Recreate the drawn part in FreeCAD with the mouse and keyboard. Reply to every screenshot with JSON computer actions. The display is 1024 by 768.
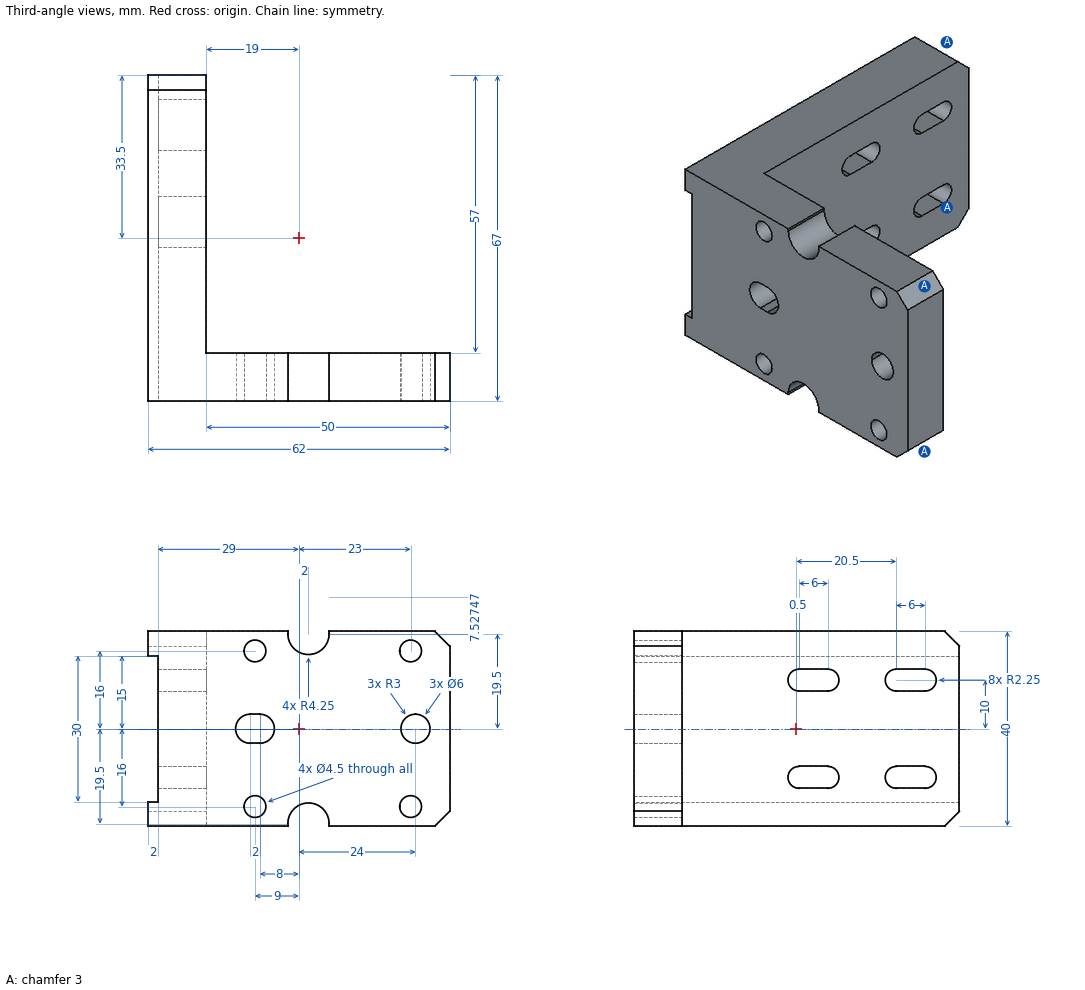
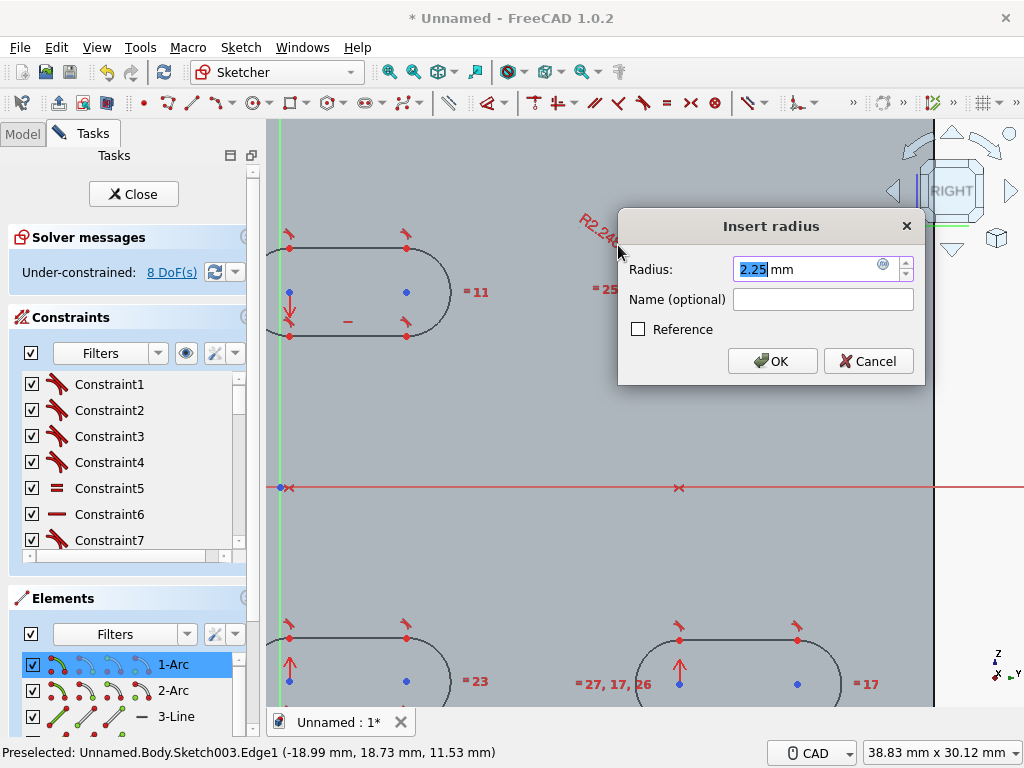
{"action": "type", "text": "2.25"}
{"action": "key", "text": "Return"}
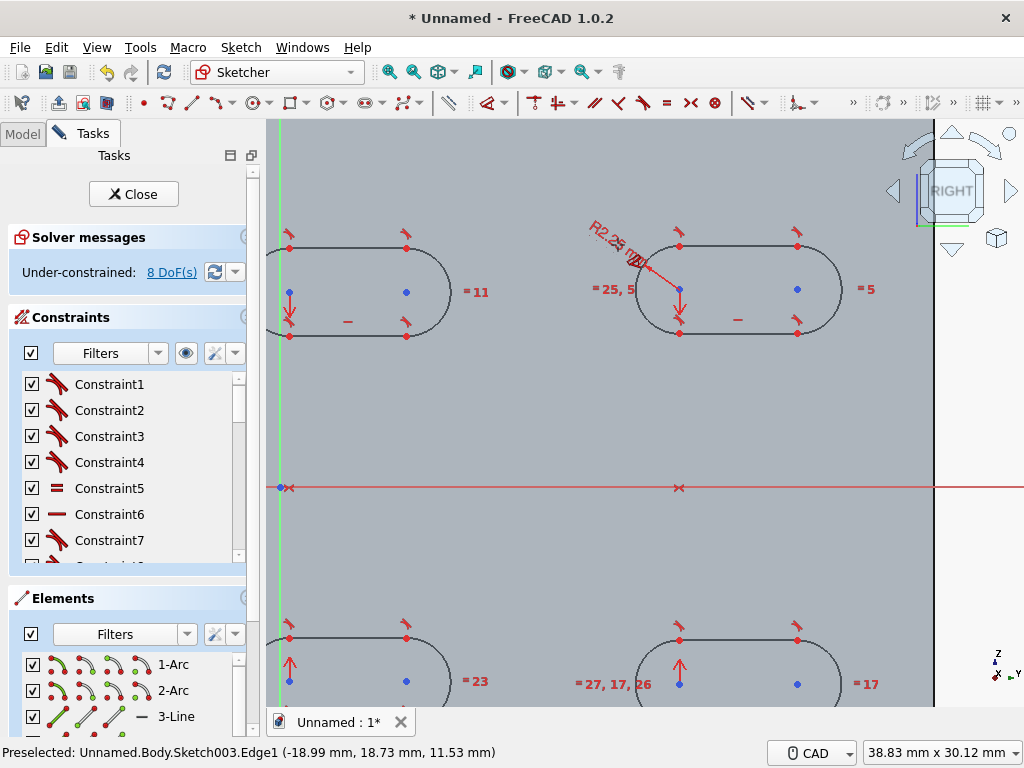
{"action": "left_click", "coordinate": [715, 246]}
{"action": "left_click", "coordinate": [739, 212]}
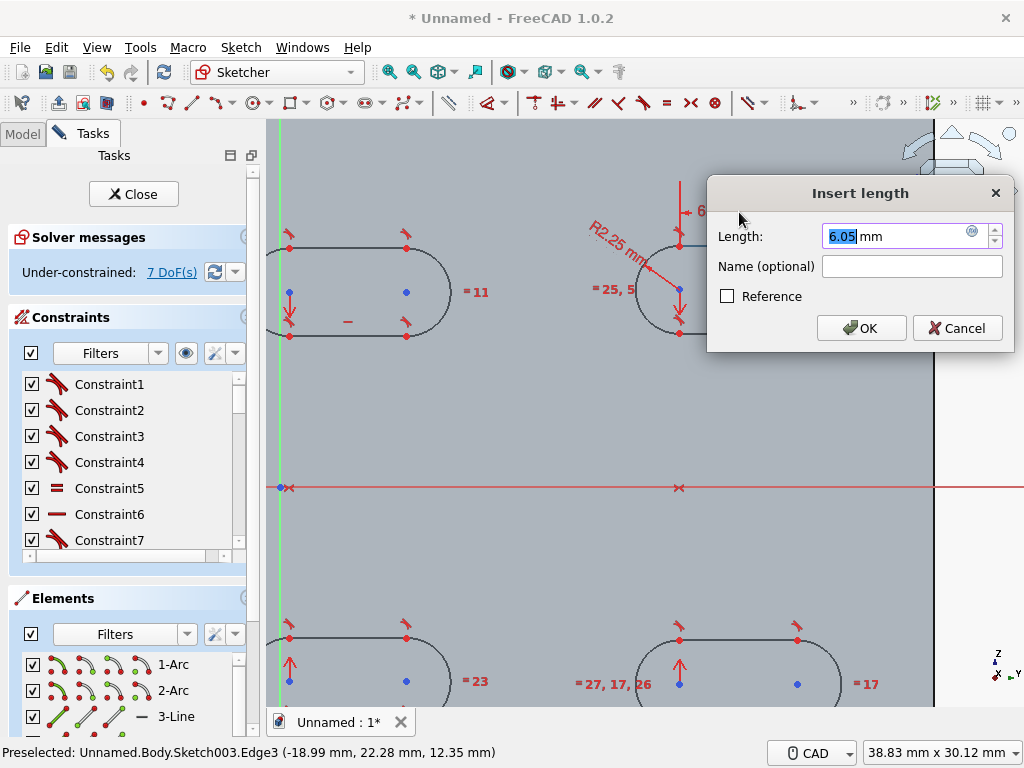
{"action": "type", "text": "6"}
{"action": "key", "text": "Return"}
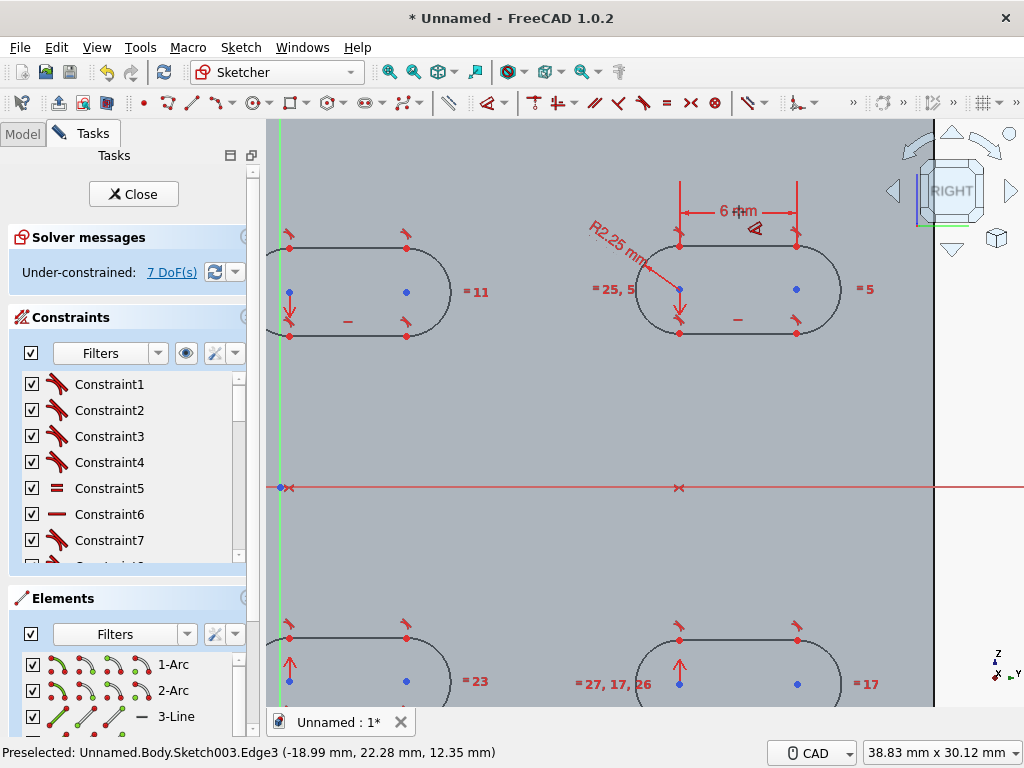
{"action": "left_click", "coordinate": [325, 248]}
{"action": "left_click", "coordinate": [350, 214]}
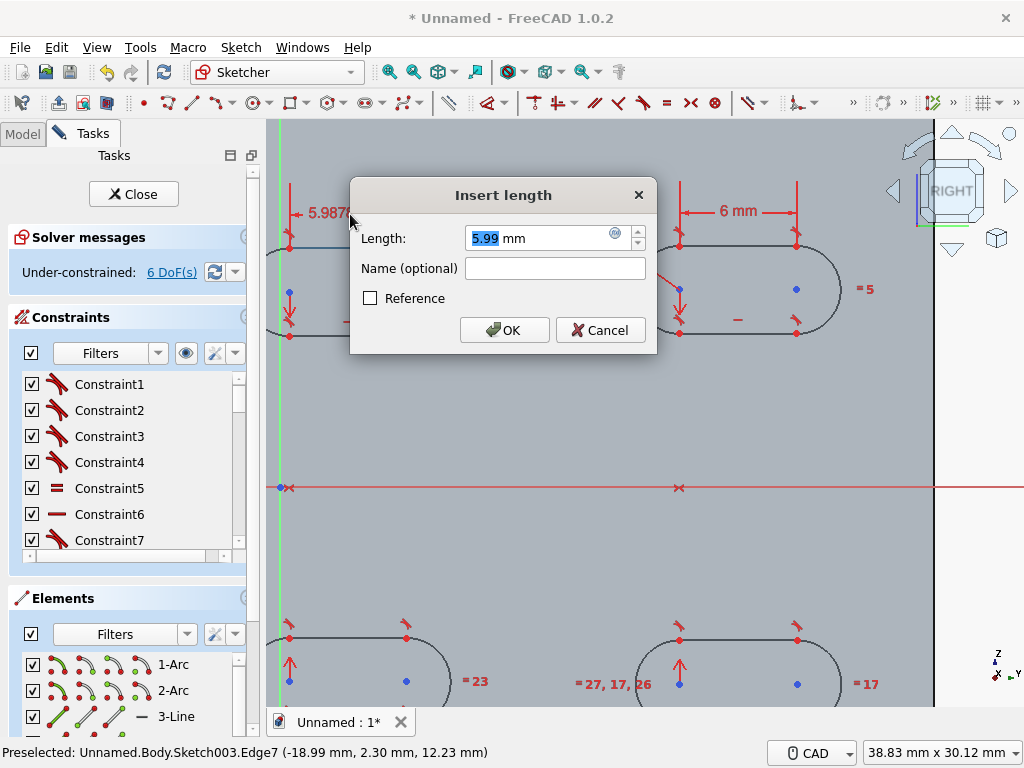
{"action": "type", "text": "6"}
{"action": "key", "text": "Return"}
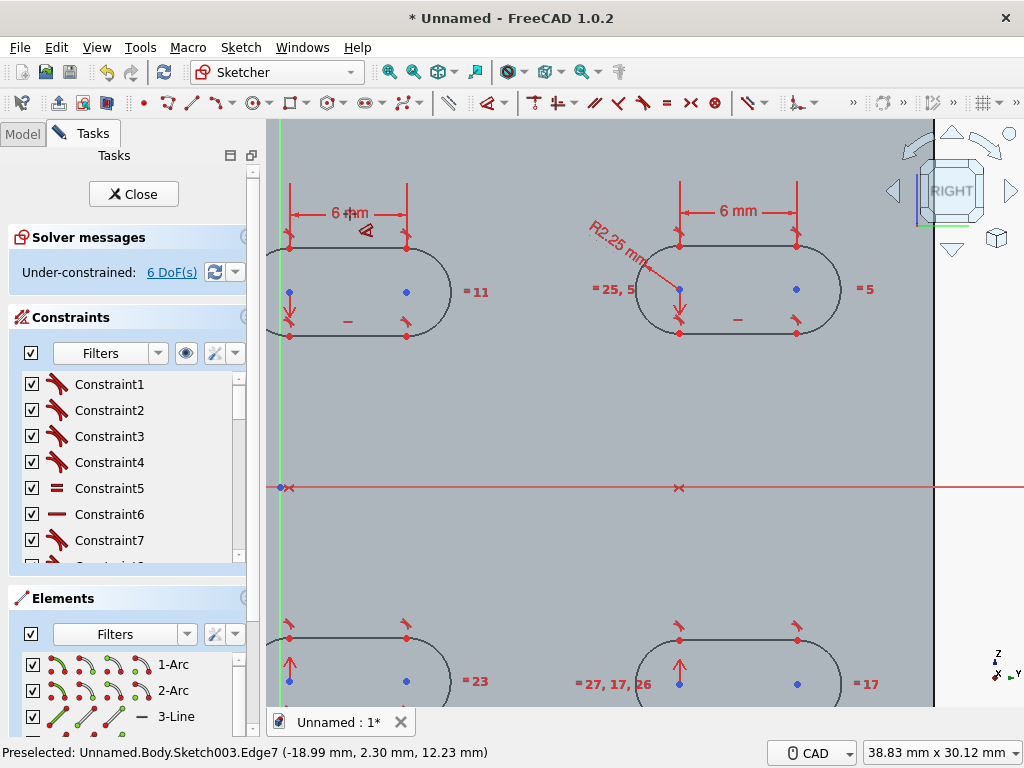
{"action": "left_click", "coordinate": [715, 640]}
{"action": "left_click", "coordinate": [739, 674]}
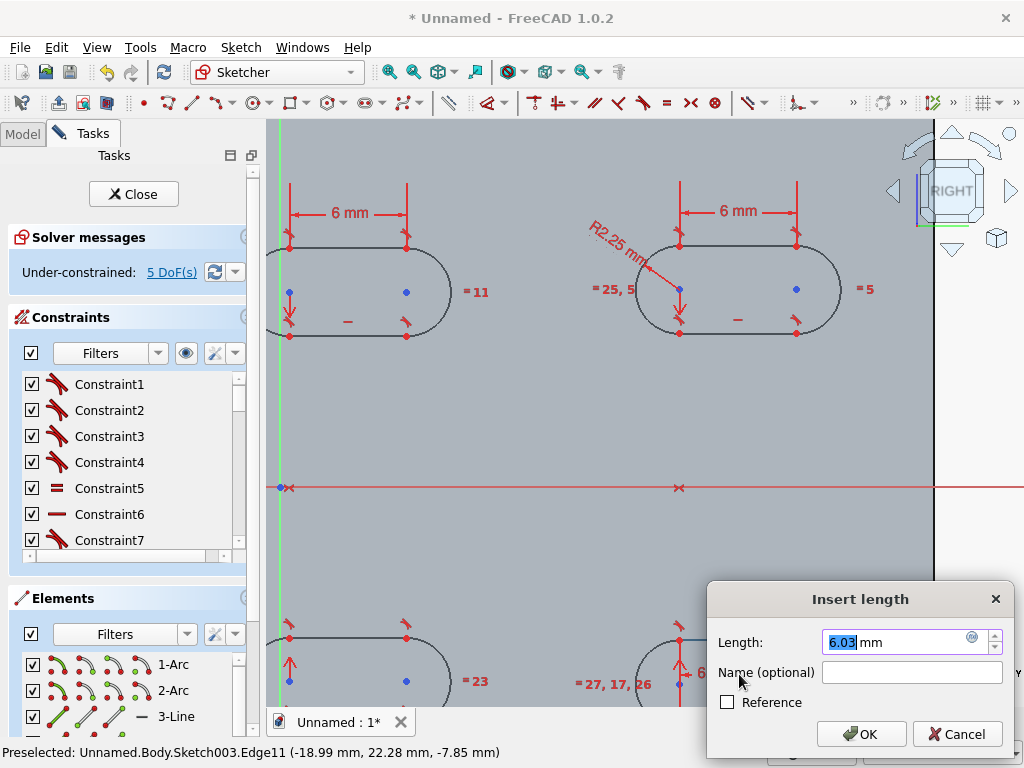
{"action": "type", "text": "6"}
{"action": "key", "text": "Return"}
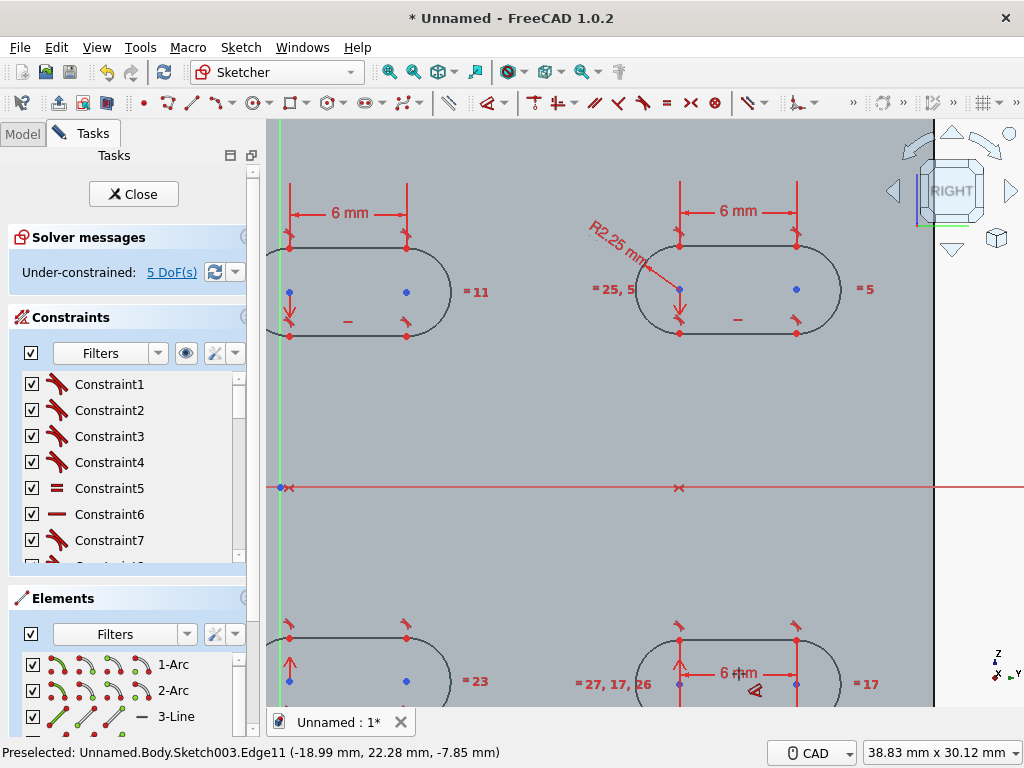
{"action": "left_click", "coordinate": [325, 638]}
{"action": "left_click", "coordinate": [350, 672]}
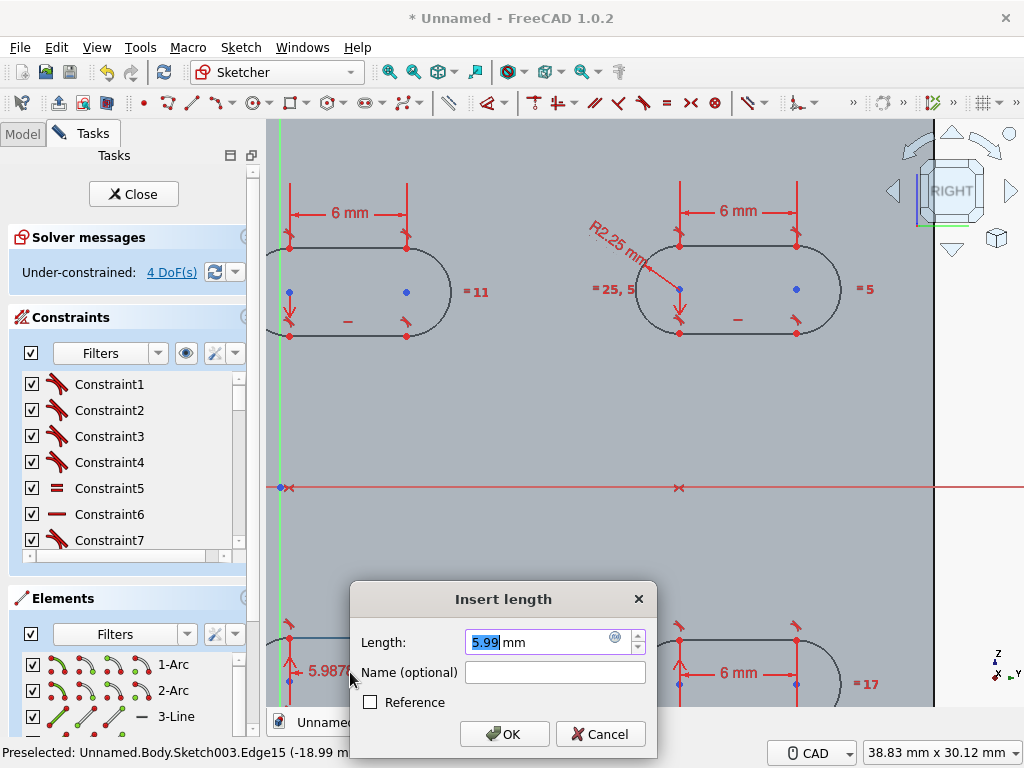
{"action": "type", "text": "6"}
{"action": "key", "text": "Return"}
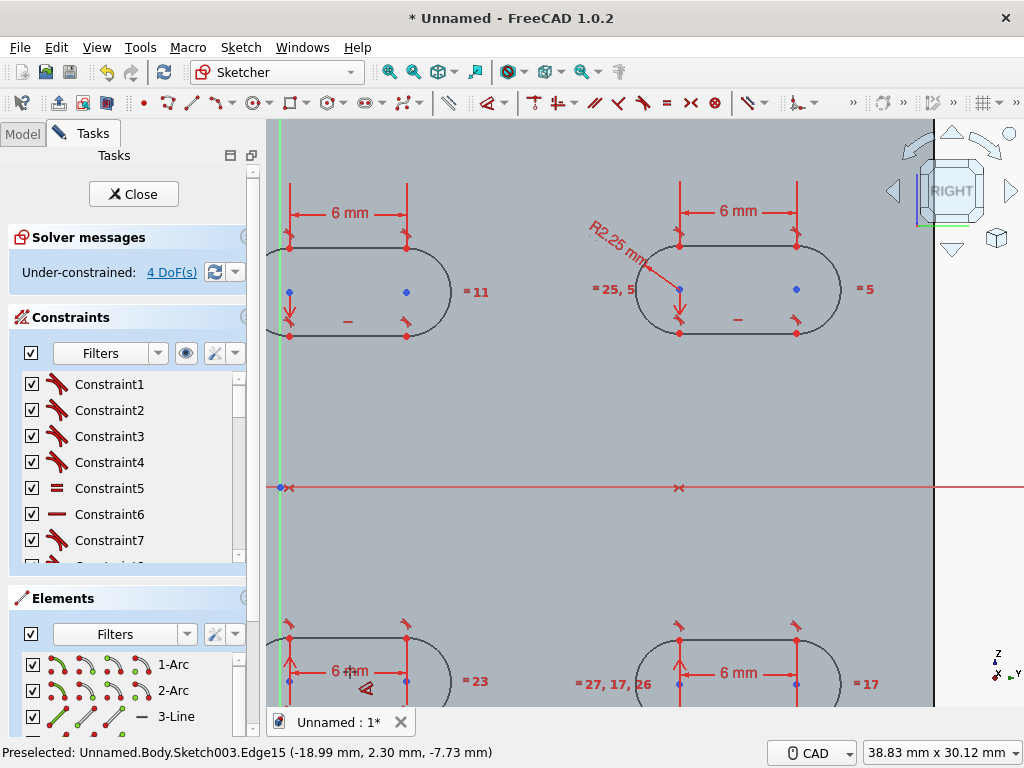
{"action": "left_click", "coordinate": [680, 290]}
{"action": "left_click", "coordinate": [714, 389]}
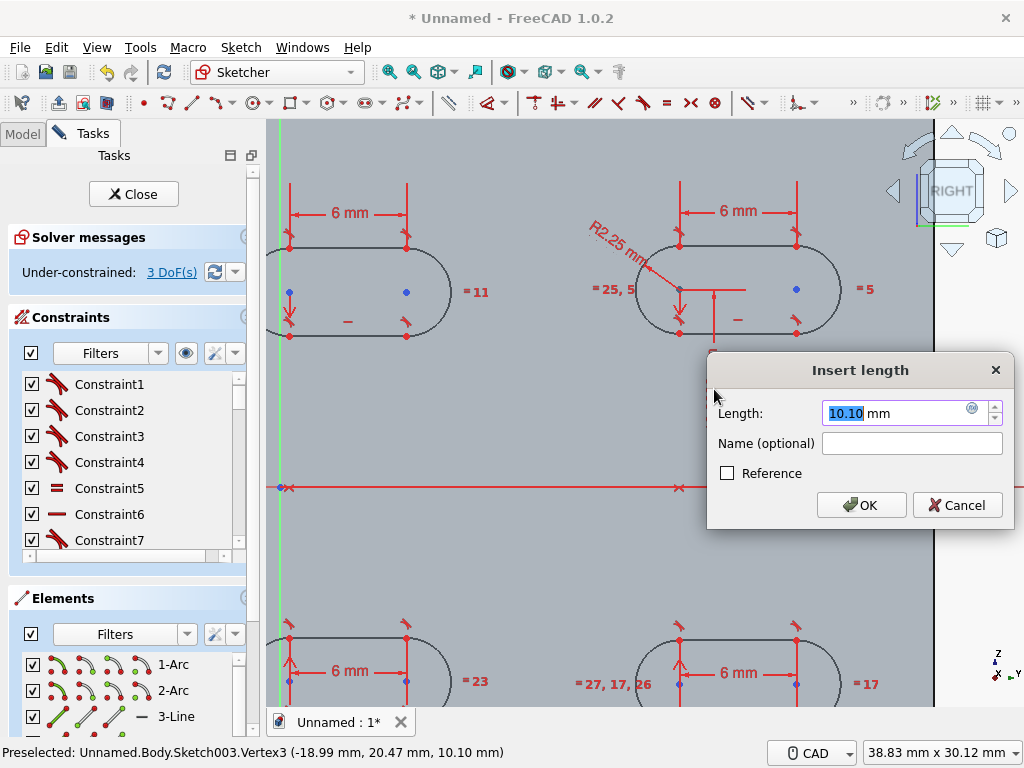
{"action": "type", "text": "10"}
{"action": "key", "text": "Return"}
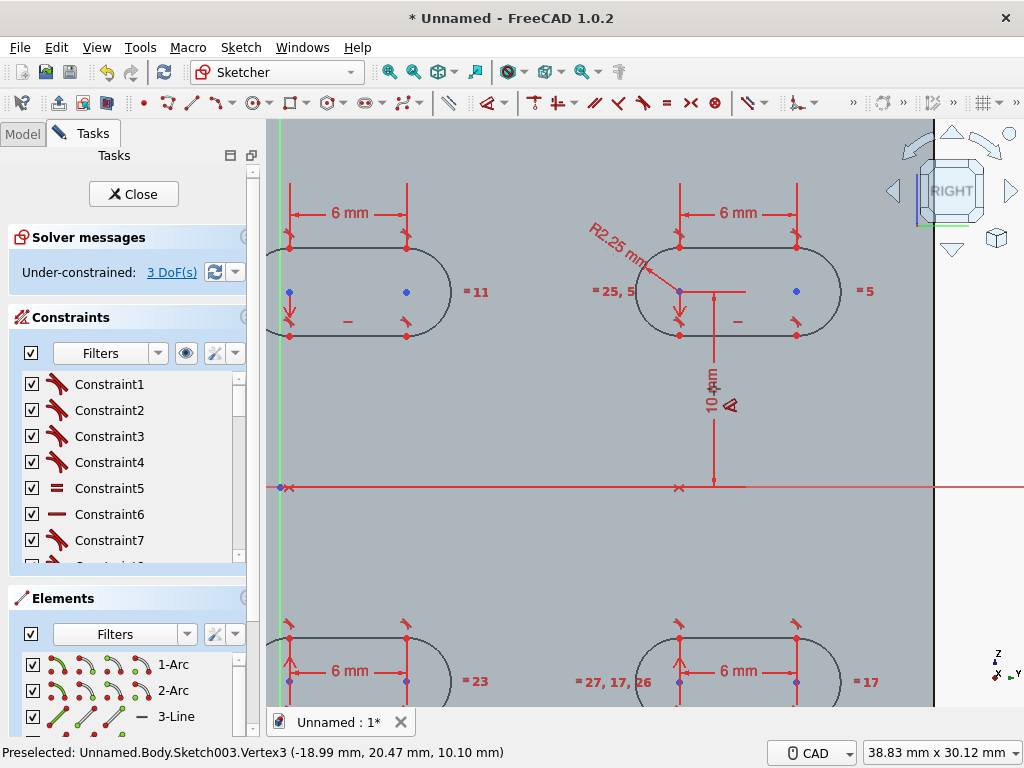
{"action": "scroll", "coordinate": [643, 262], "scroll_direction": "down", "scroll_amount": 2}